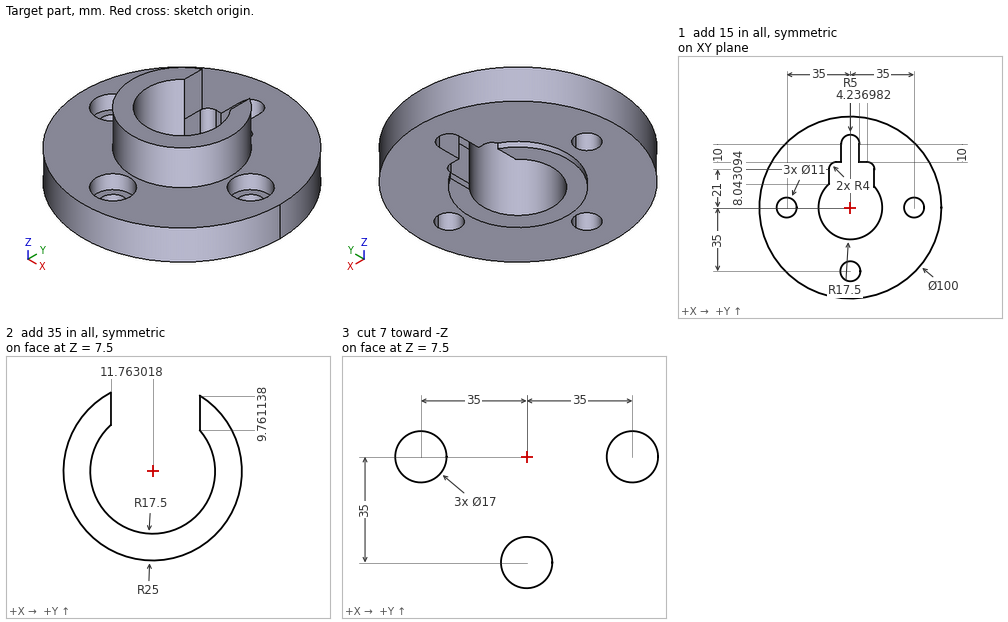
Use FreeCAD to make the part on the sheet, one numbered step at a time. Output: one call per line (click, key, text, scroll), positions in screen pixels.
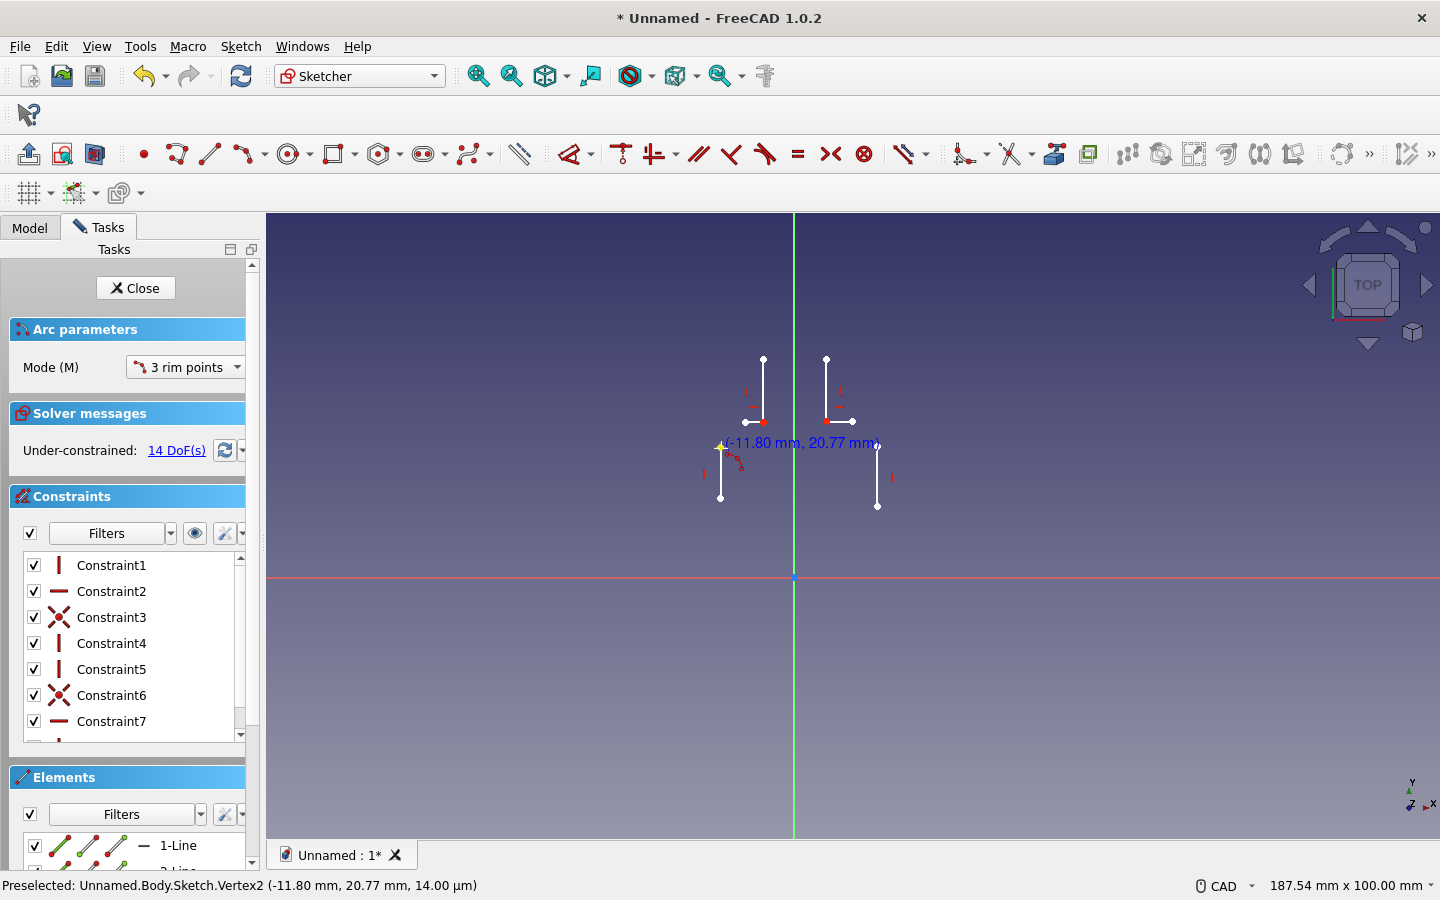
scroll(746, 421, up, 4)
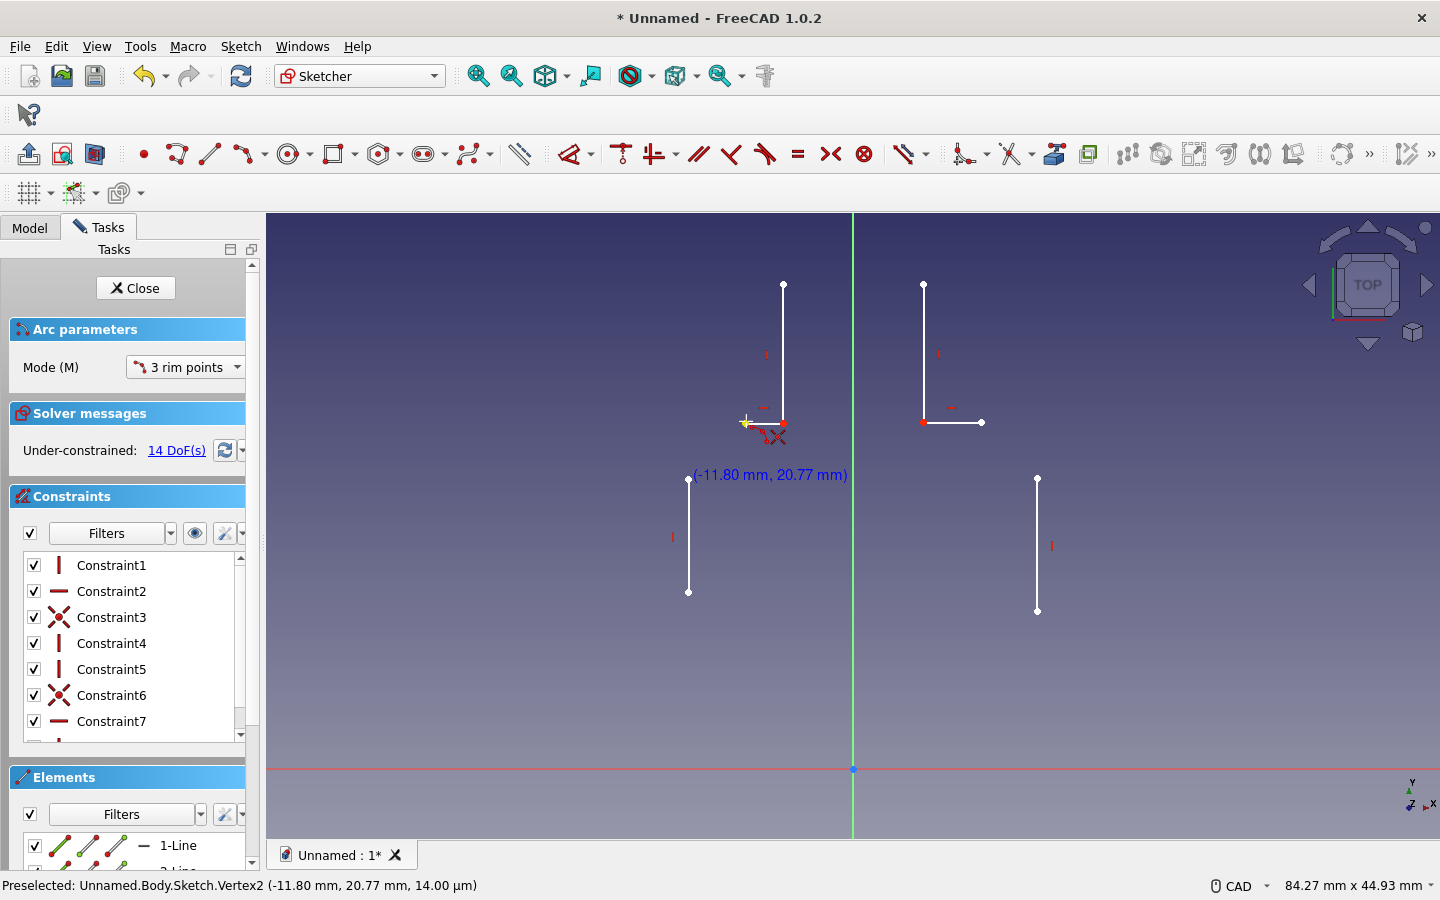
click(745, 424)
click(706, 437)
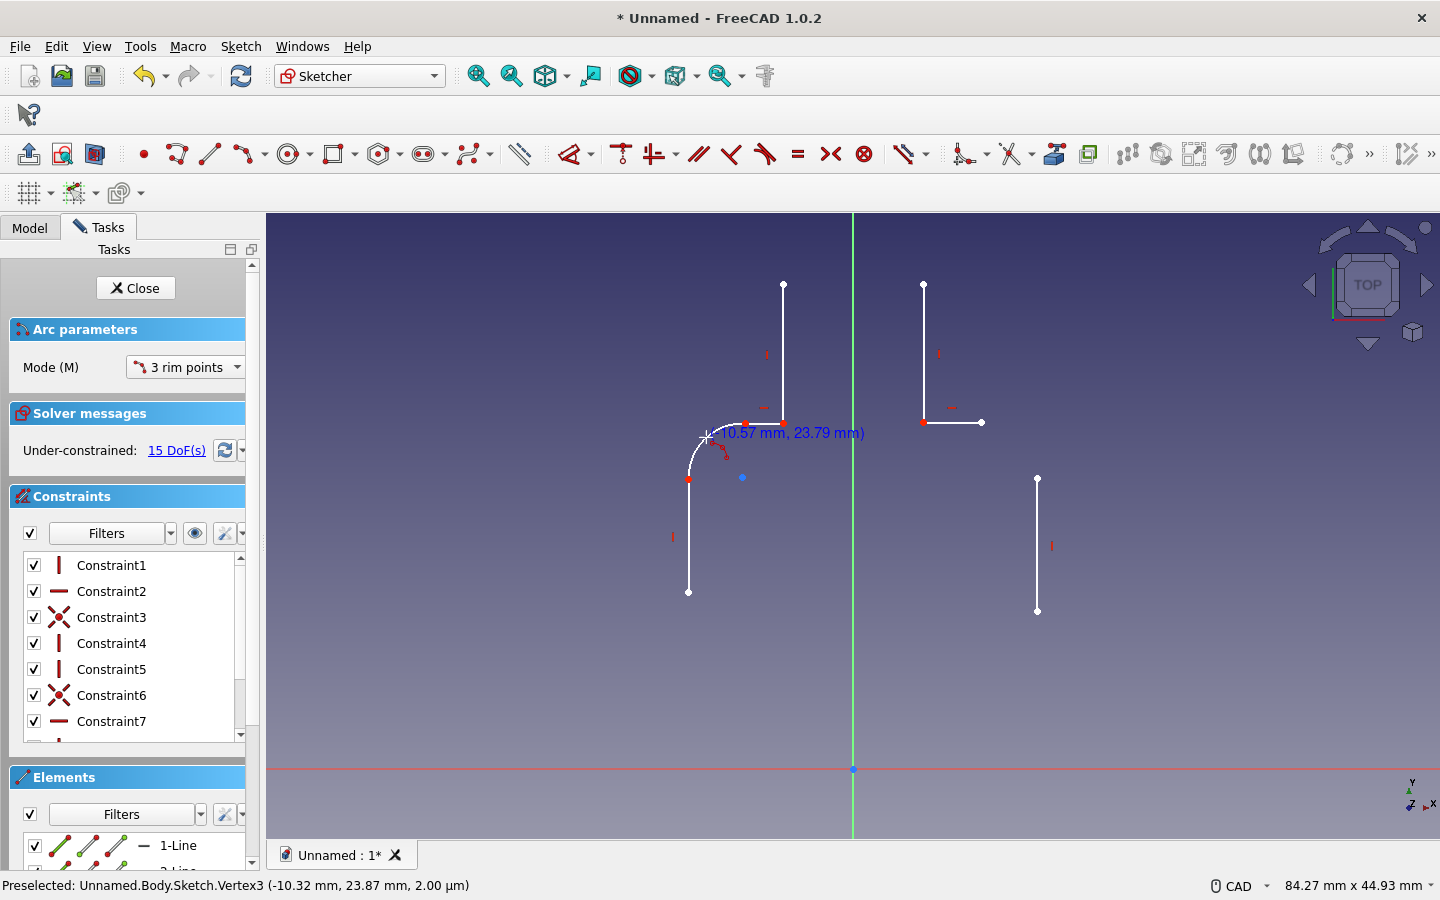
click(783, 285)
click(924, 285)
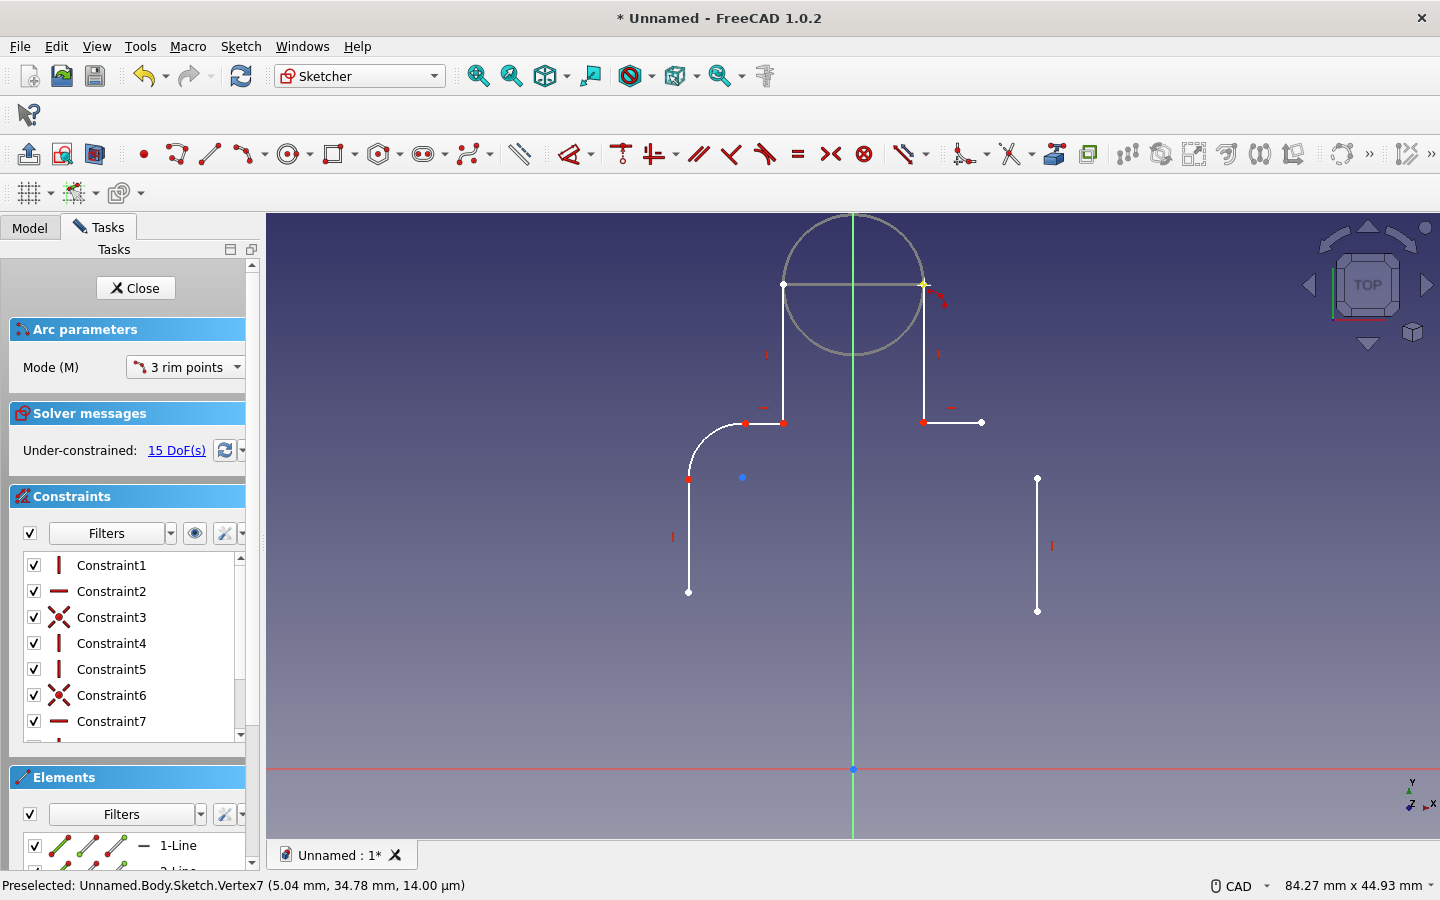
scroll(755, 421, down, 6)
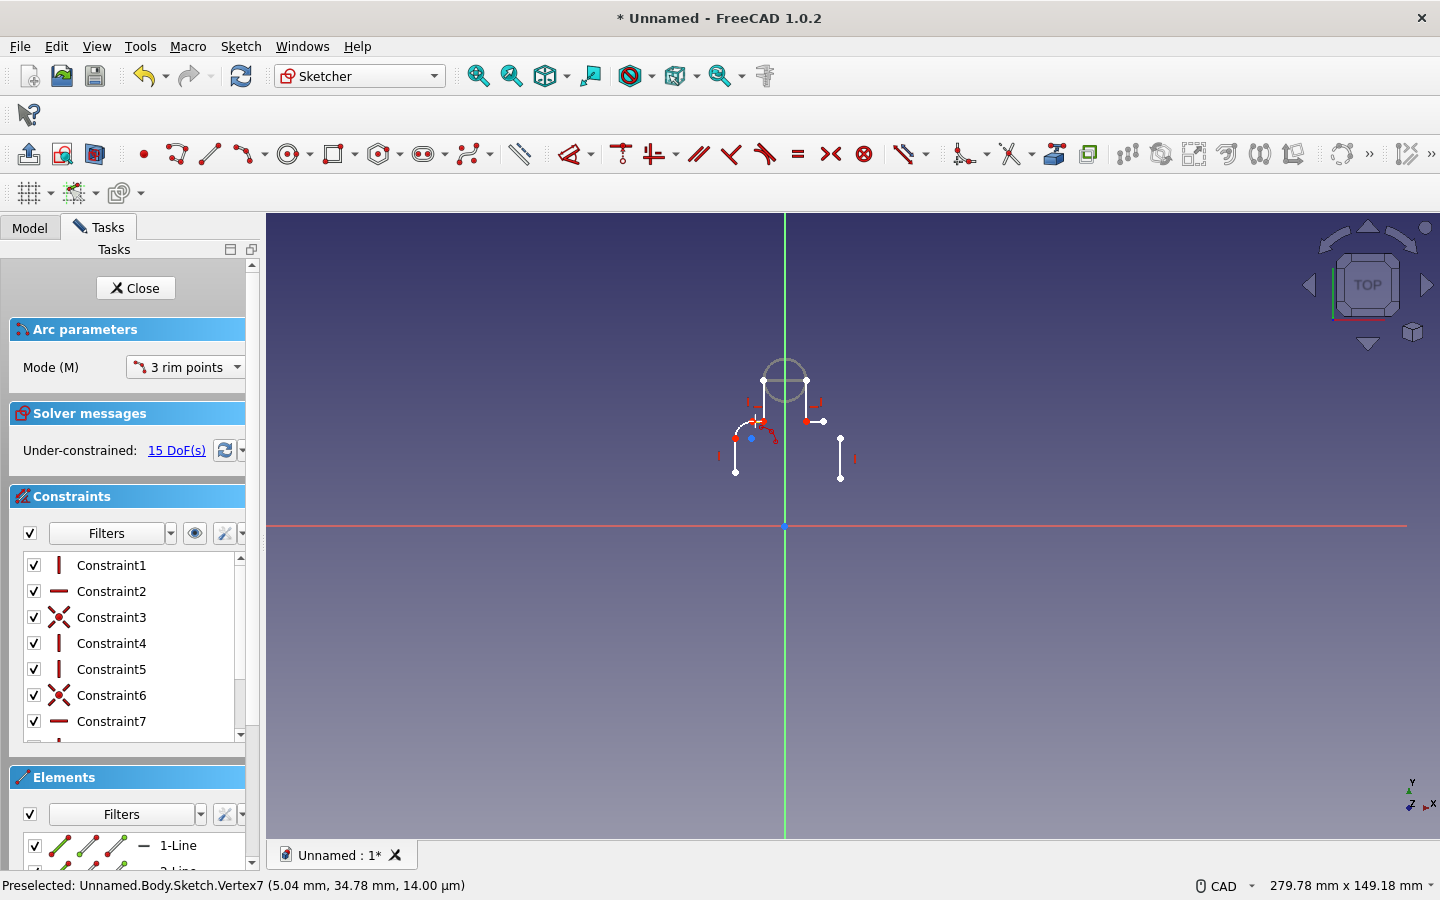
scroll(797, 362, up, 2)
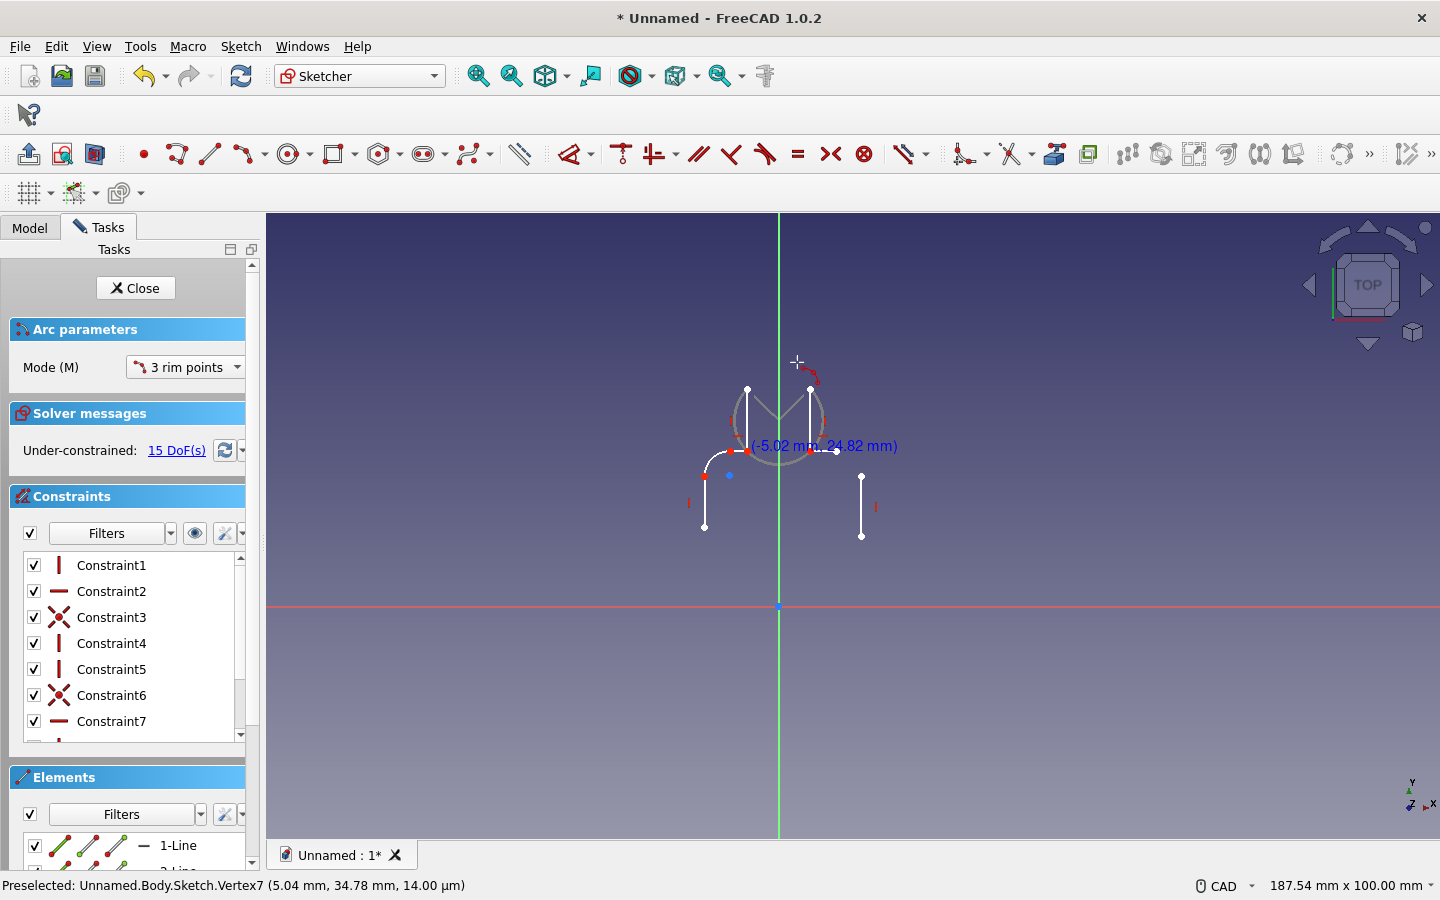
click(797, 362)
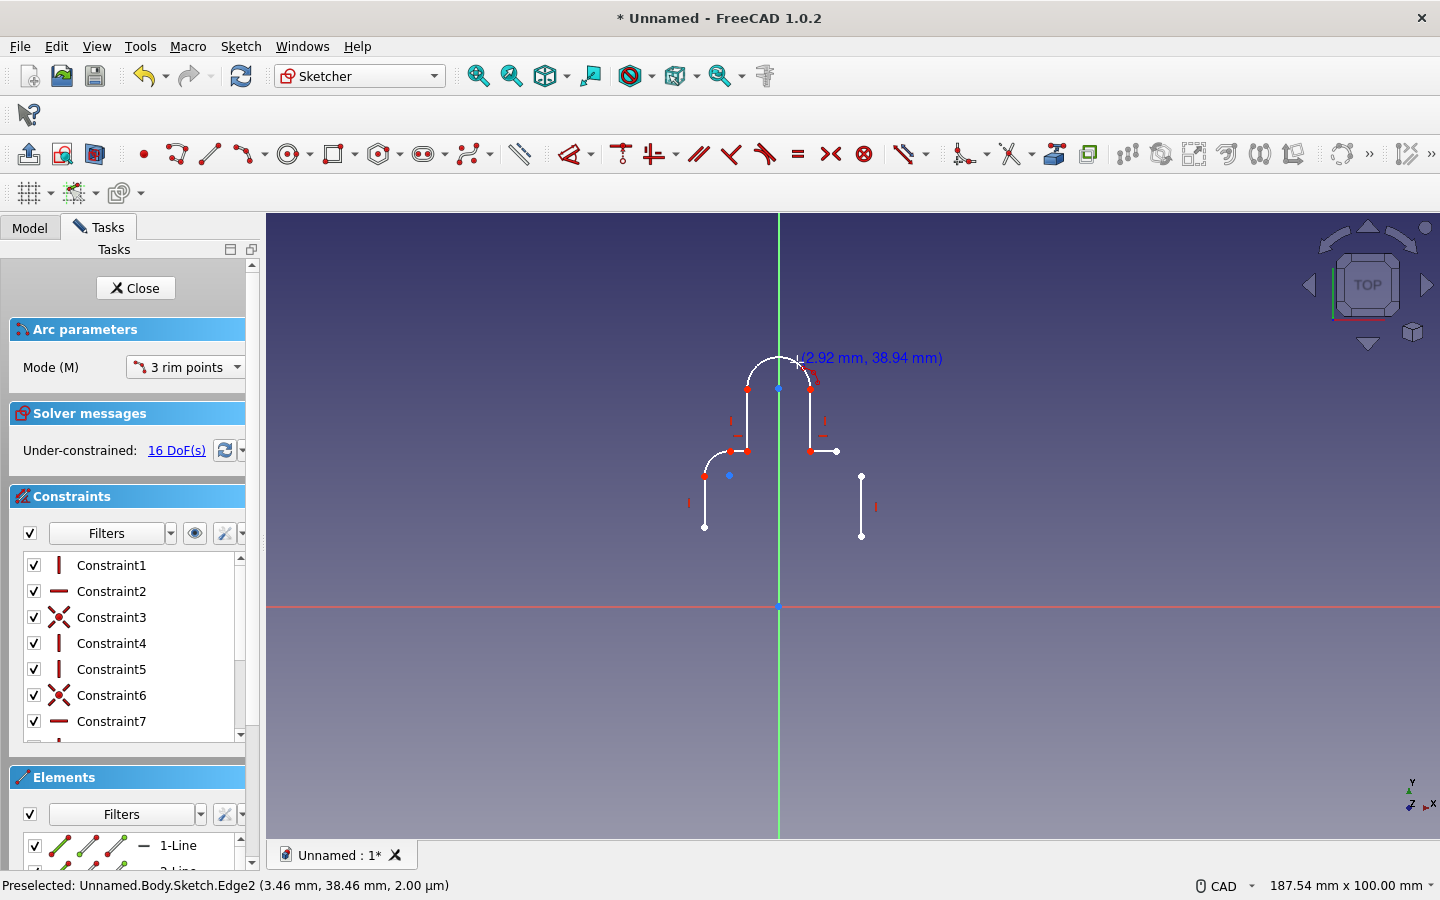
click(836, 451)
click(861, 476)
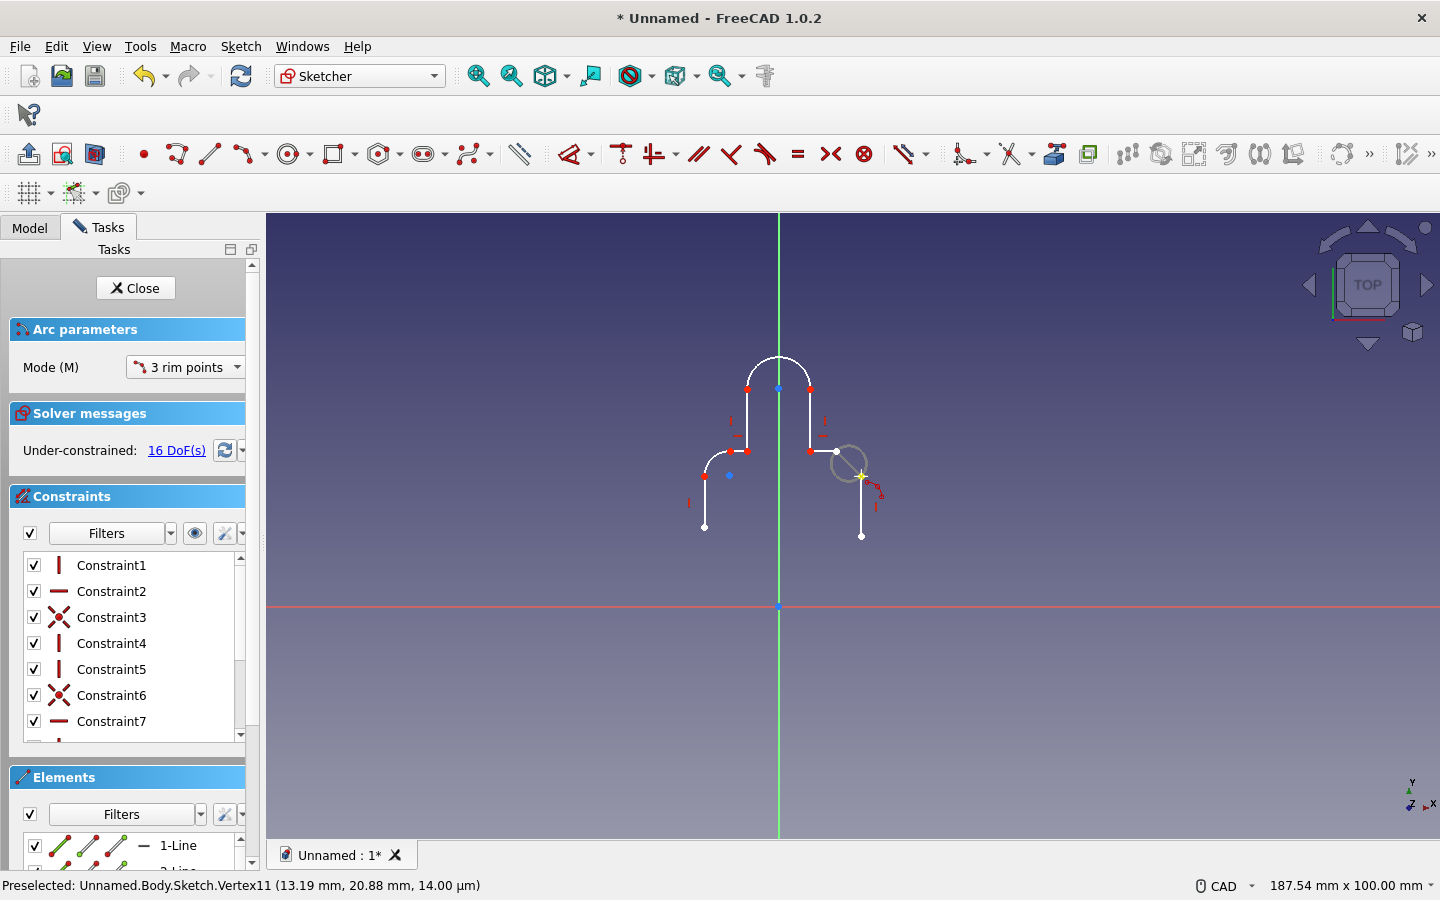
scroll(854, 458, up, 4)